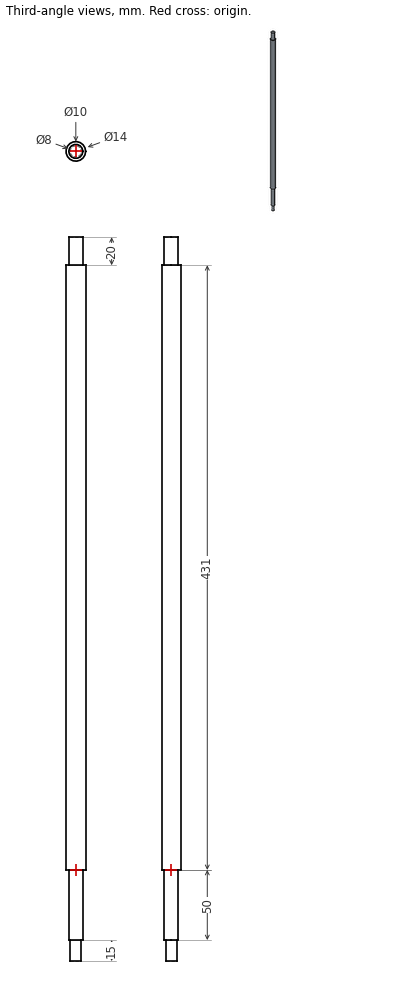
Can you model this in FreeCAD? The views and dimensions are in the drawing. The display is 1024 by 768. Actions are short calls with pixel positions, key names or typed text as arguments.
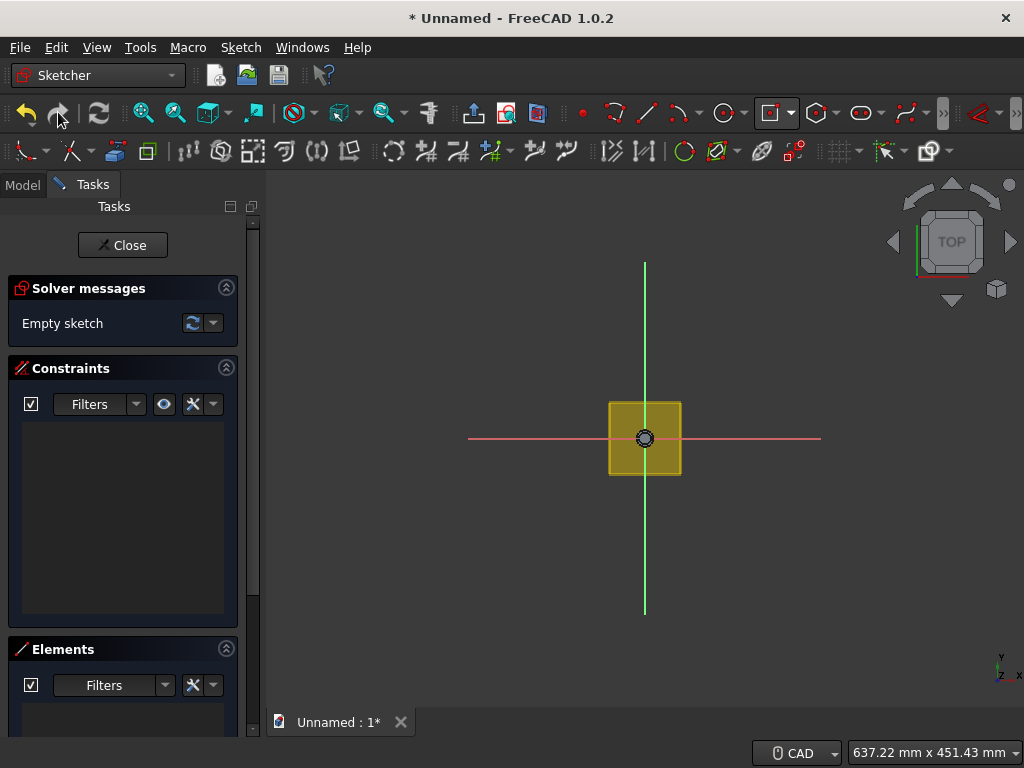
click(538, 114)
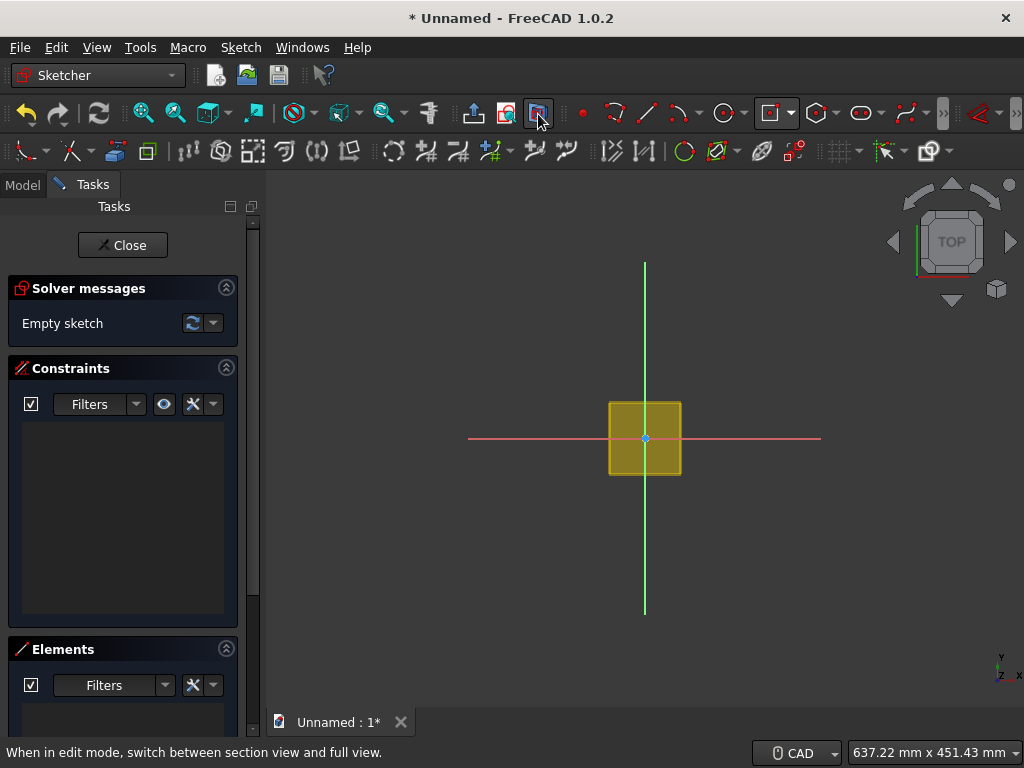
scroll(649, 438, up, 15)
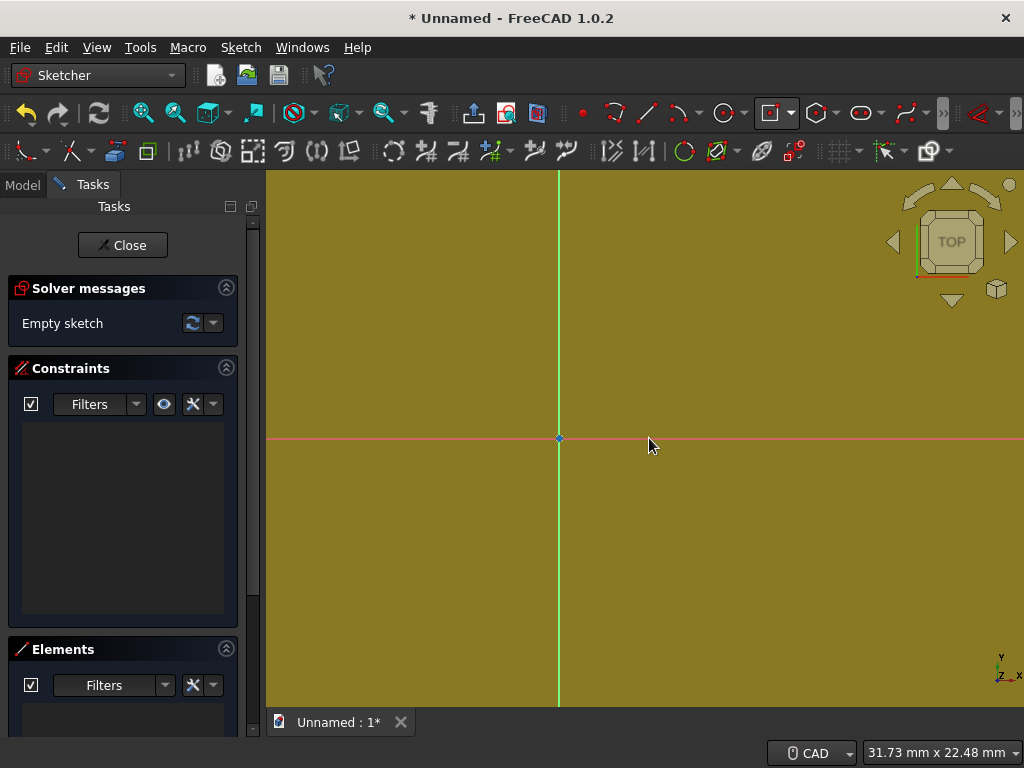
scroll(523, 439, up, 2)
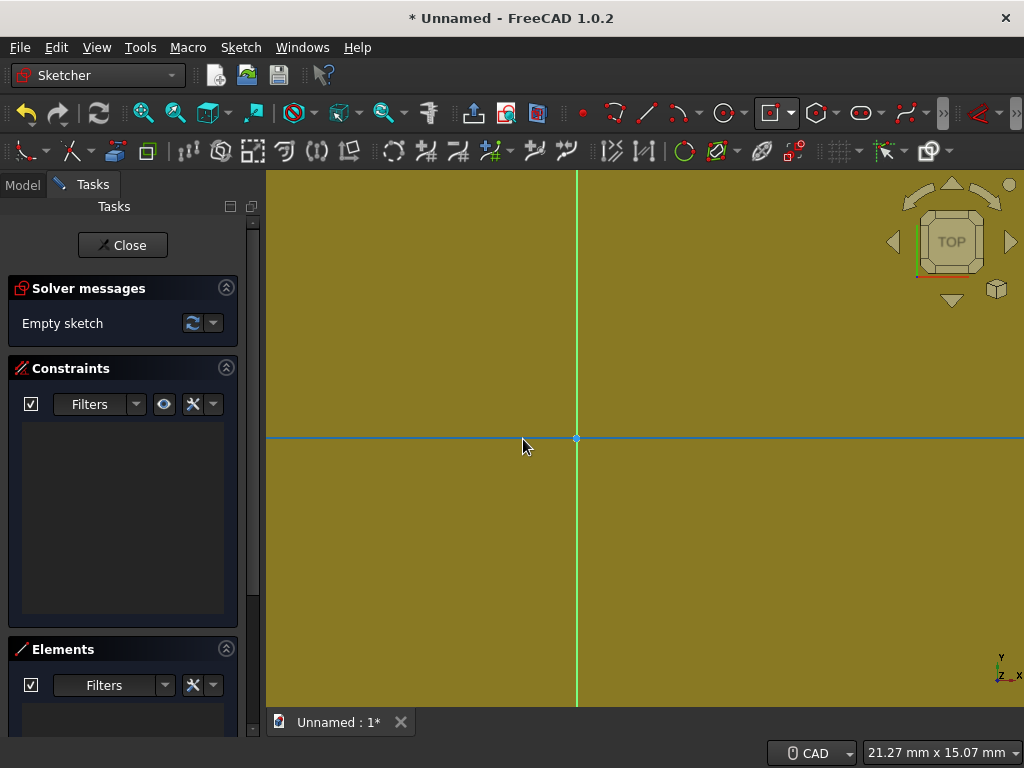
key(g)
key(c)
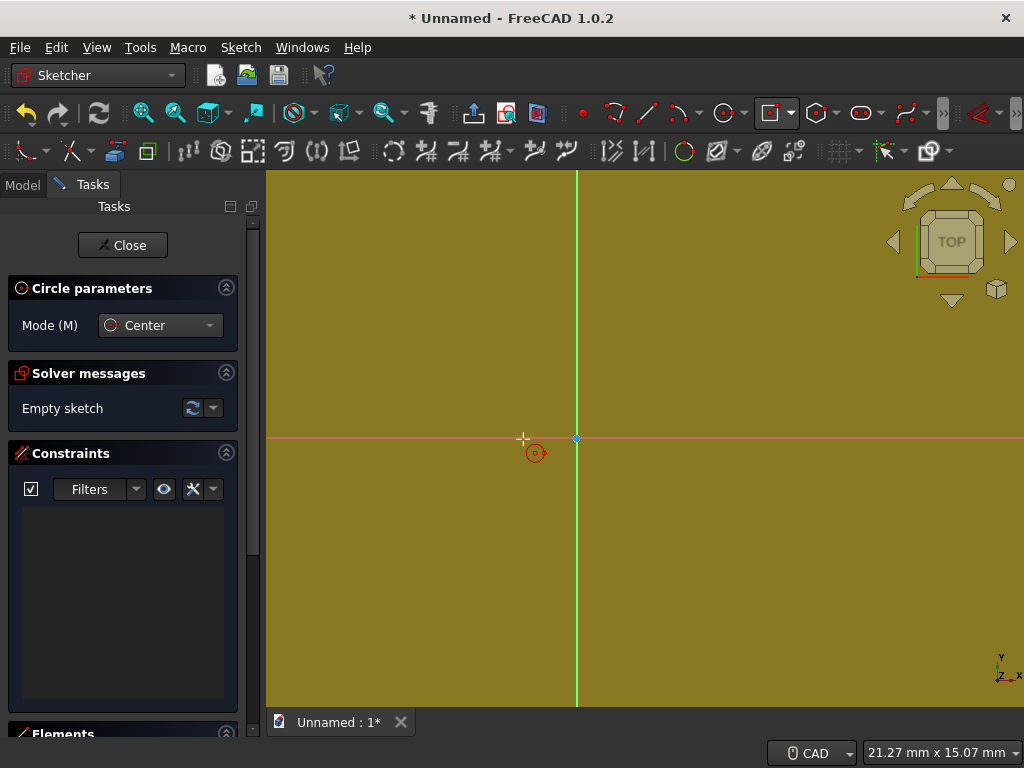
click(577, 438)
move(703, 312)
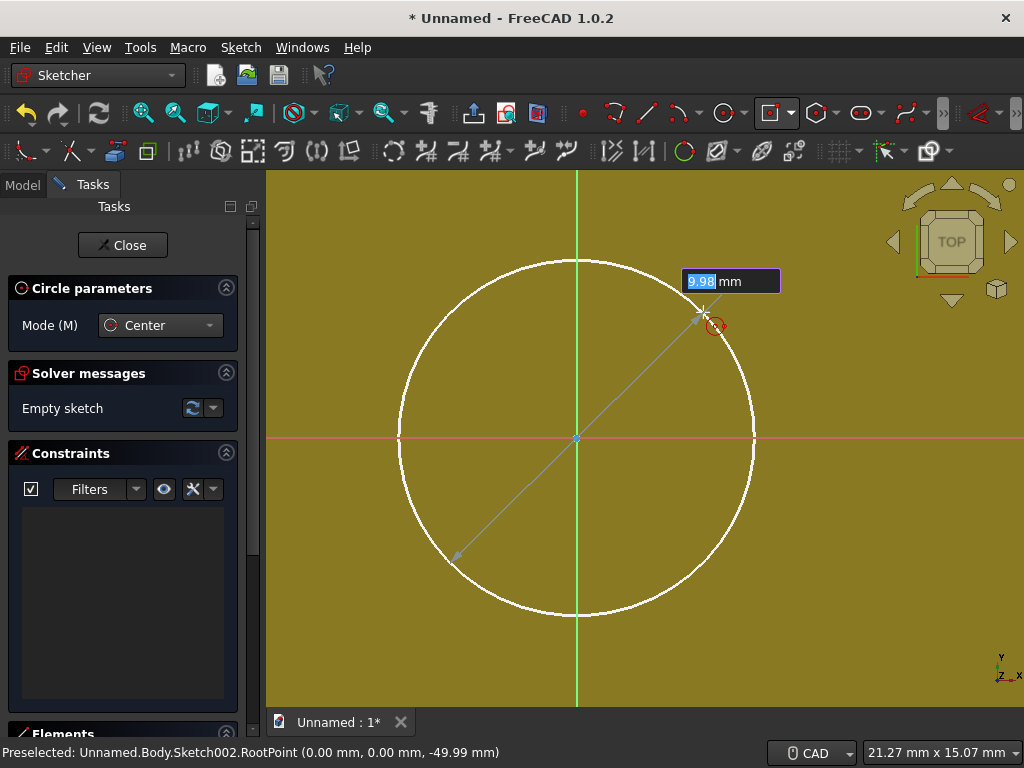
text(10)
key(Return)
key(Escape)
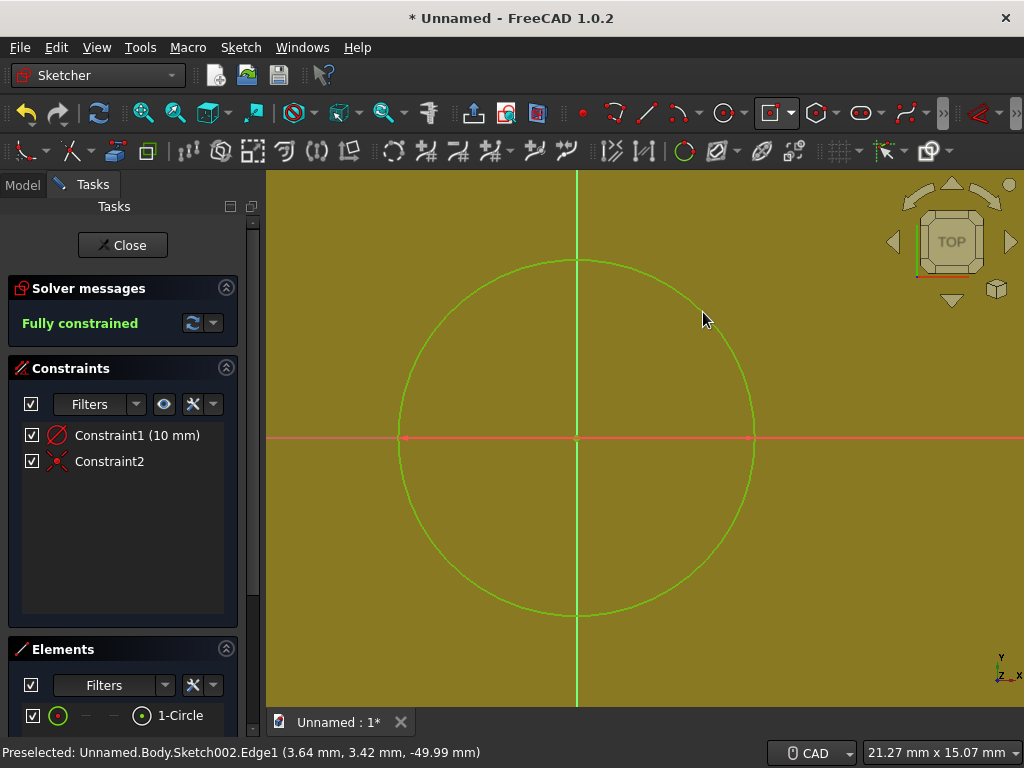
click(123, 245)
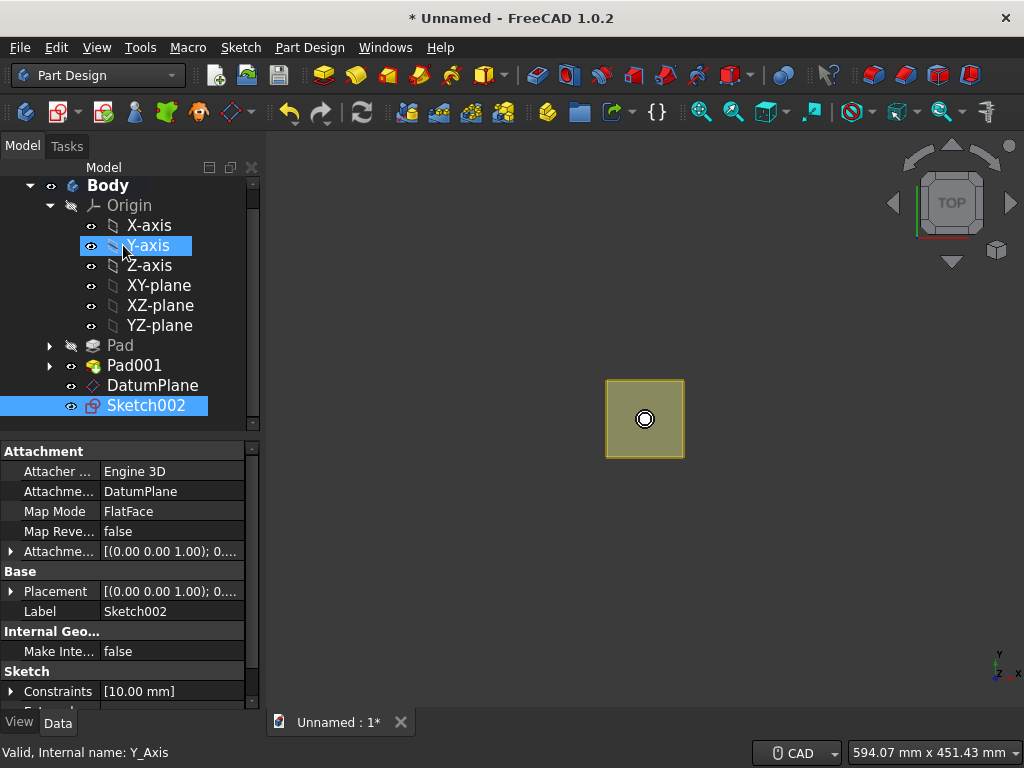
click(324, 76)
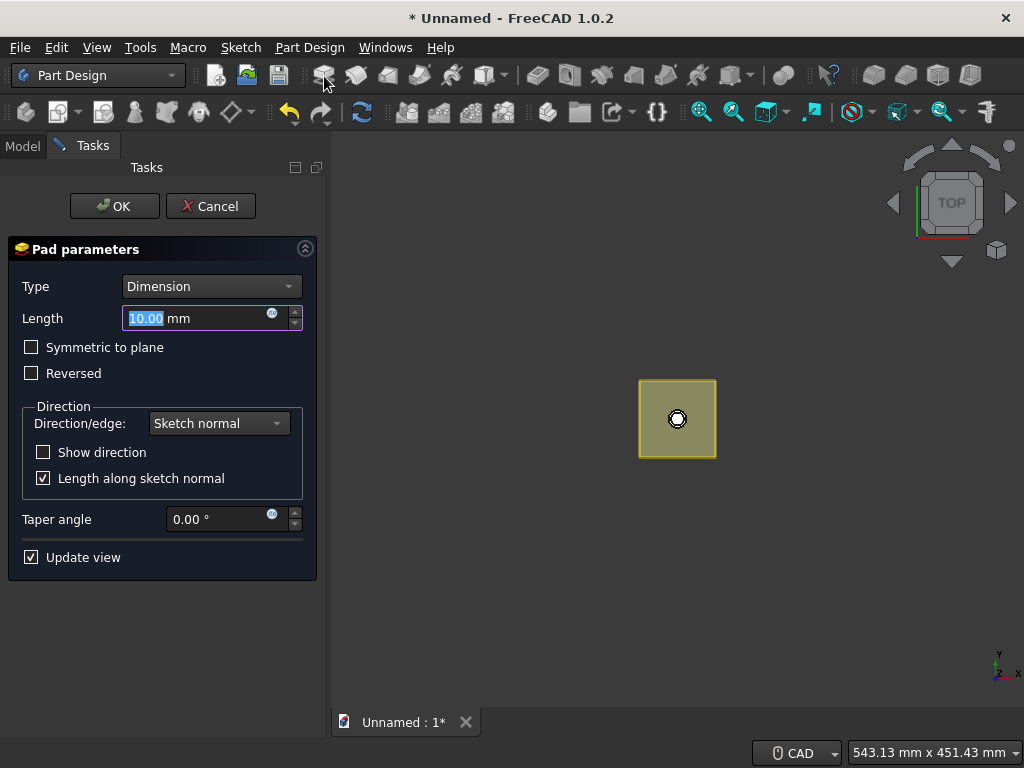
text(50)
key(Tab)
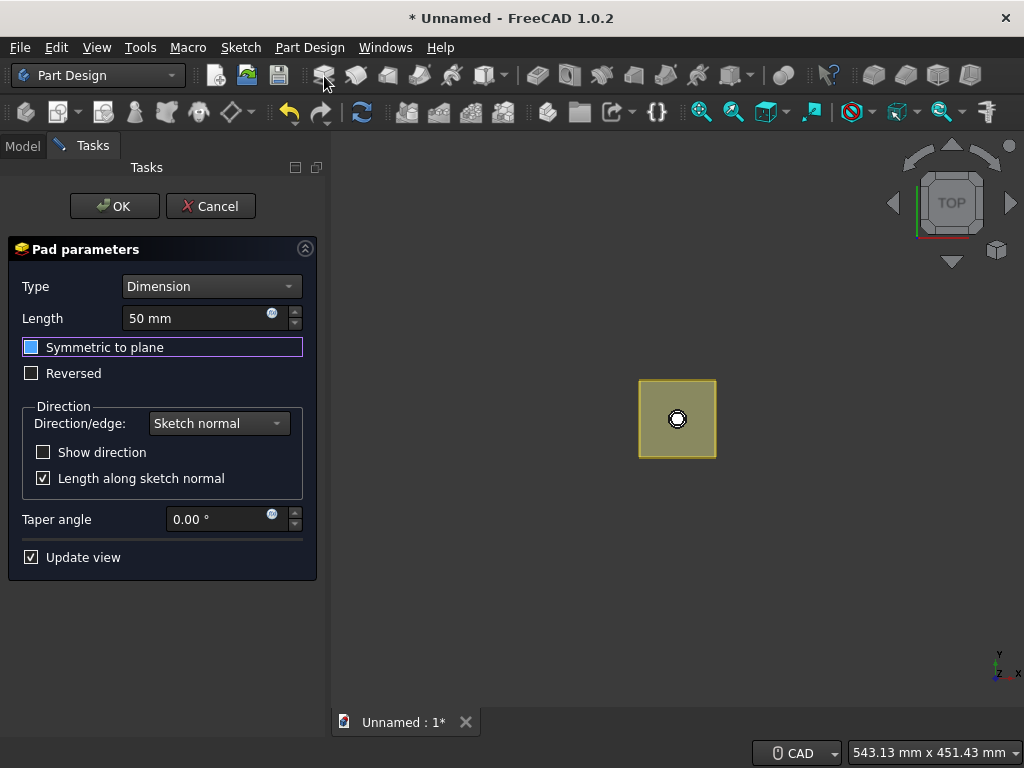
click(115, 206)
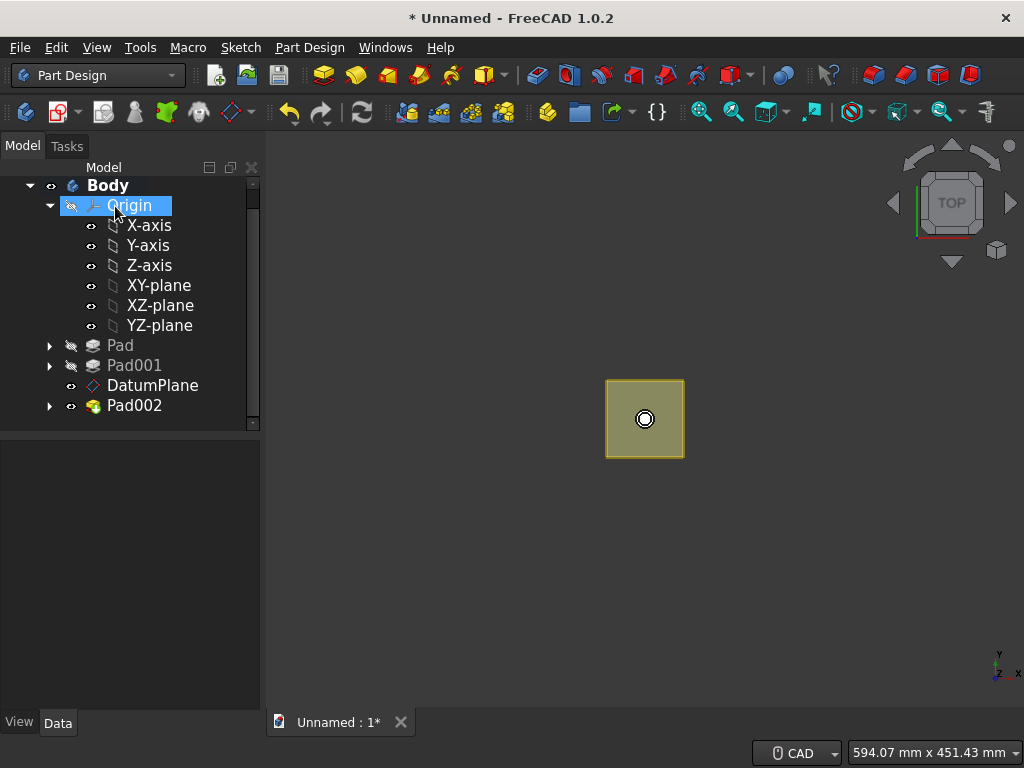
click(116, 386)
key(space)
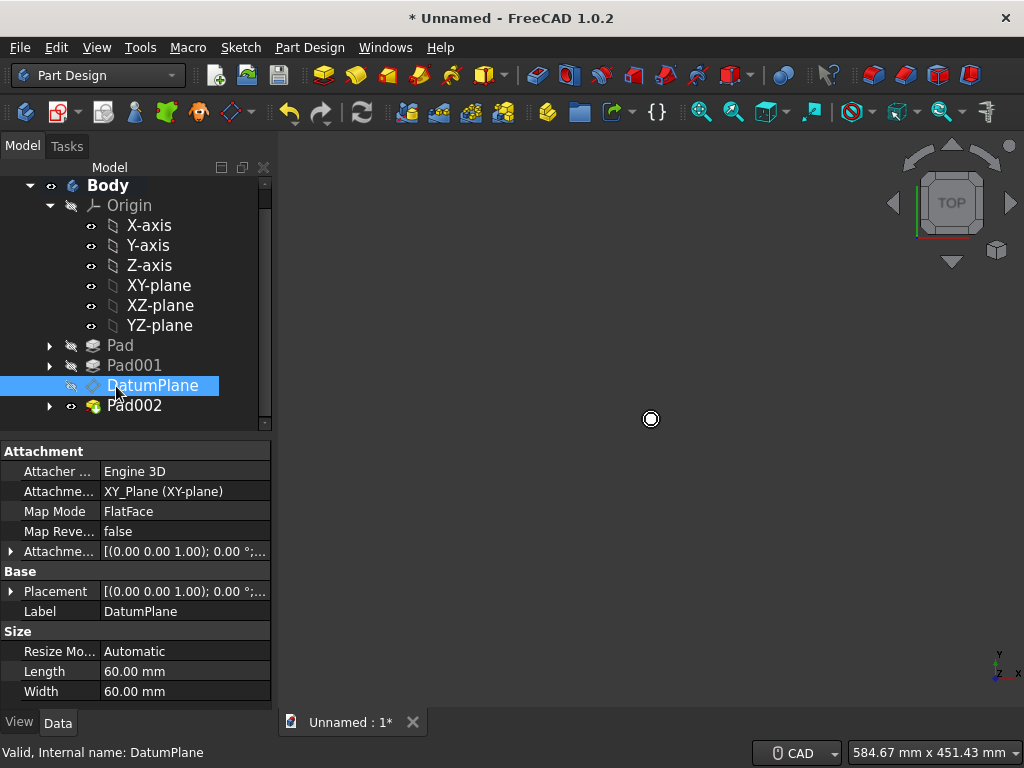
click(702, 112)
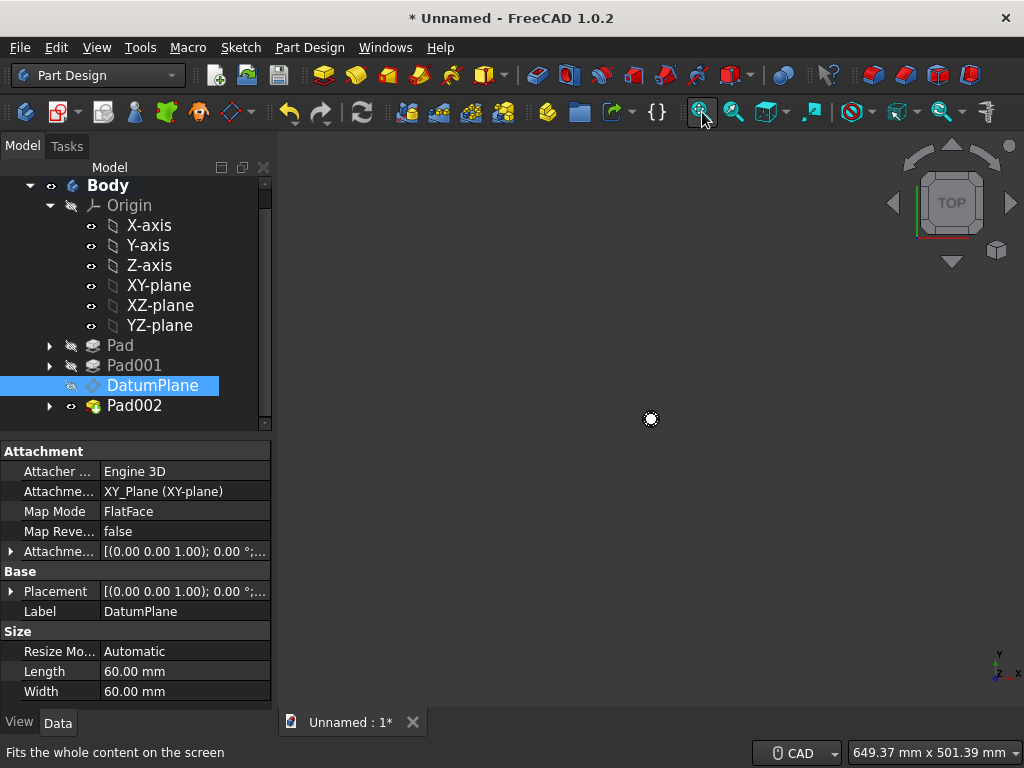
key(5)